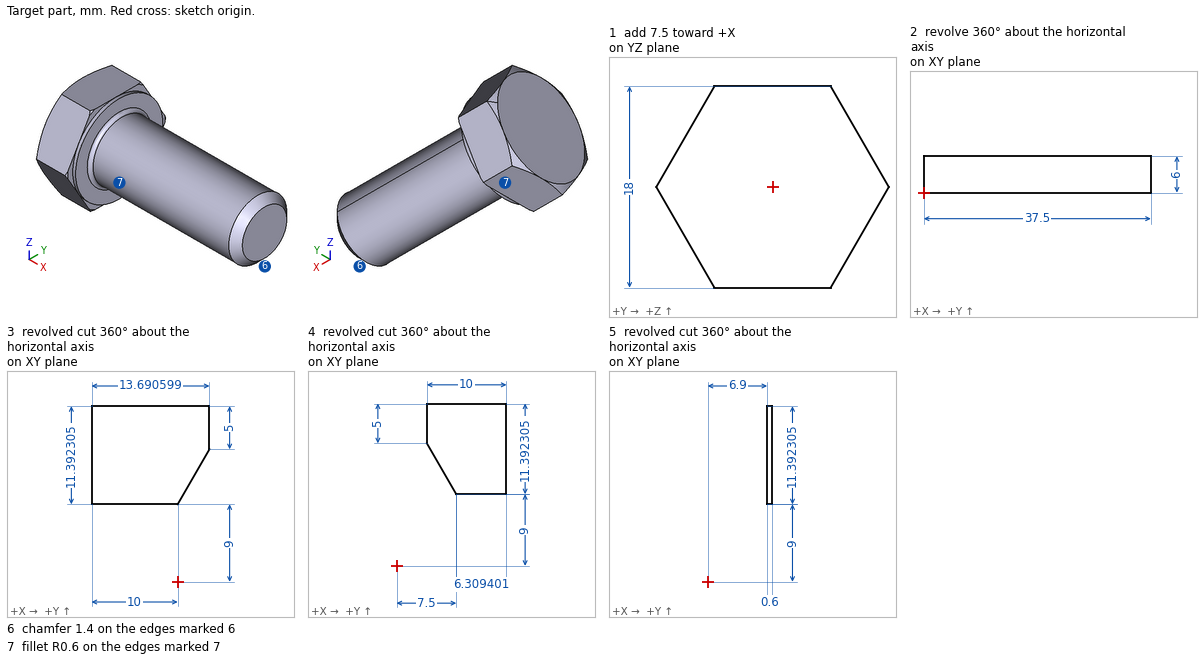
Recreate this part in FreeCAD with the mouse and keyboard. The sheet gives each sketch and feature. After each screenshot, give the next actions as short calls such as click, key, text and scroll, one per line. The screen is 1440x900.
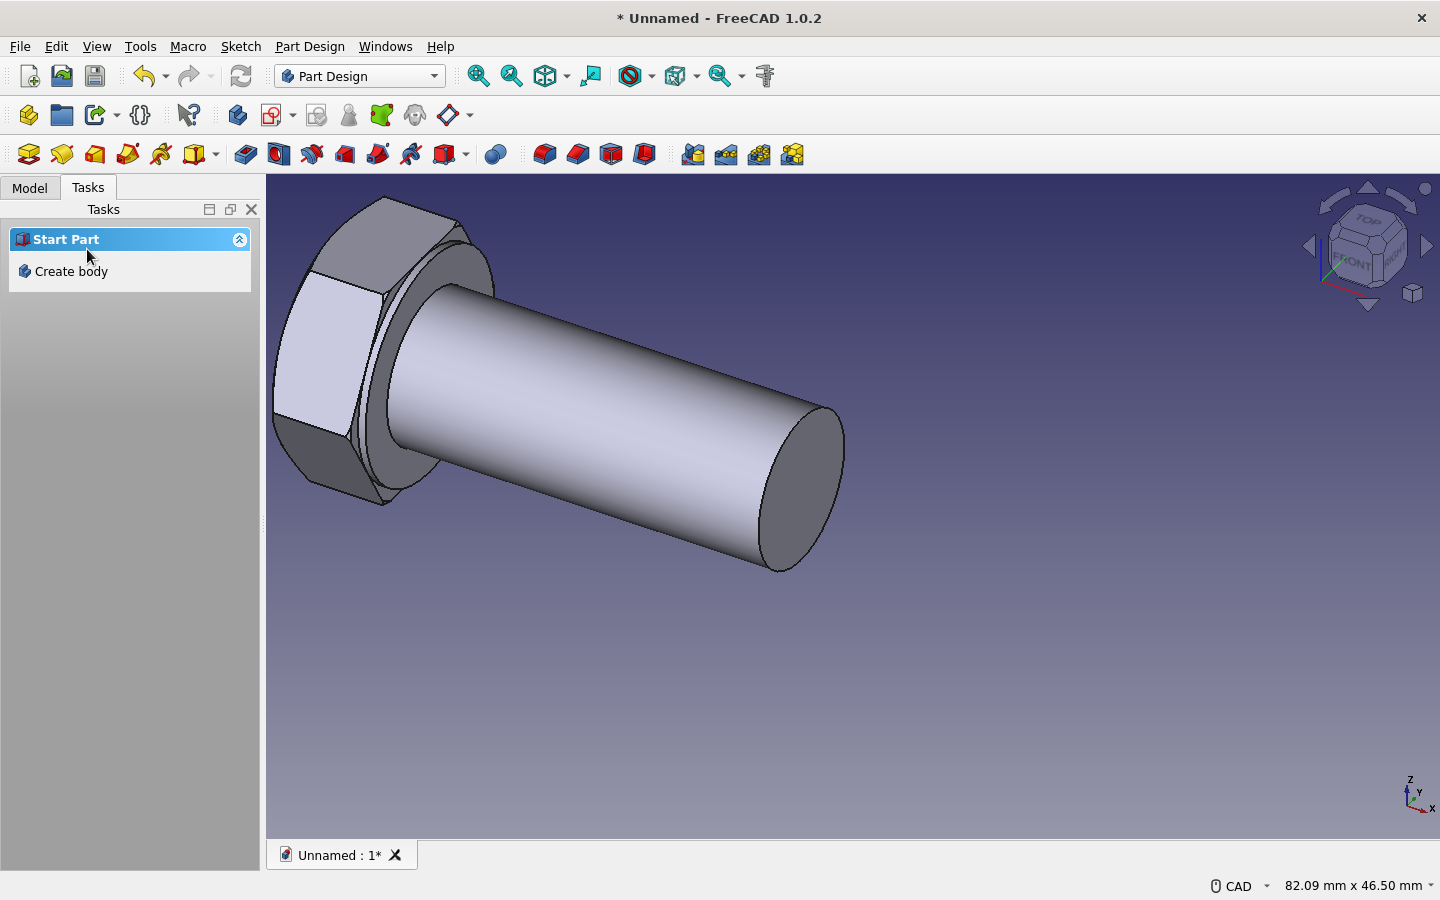
click(479, 76)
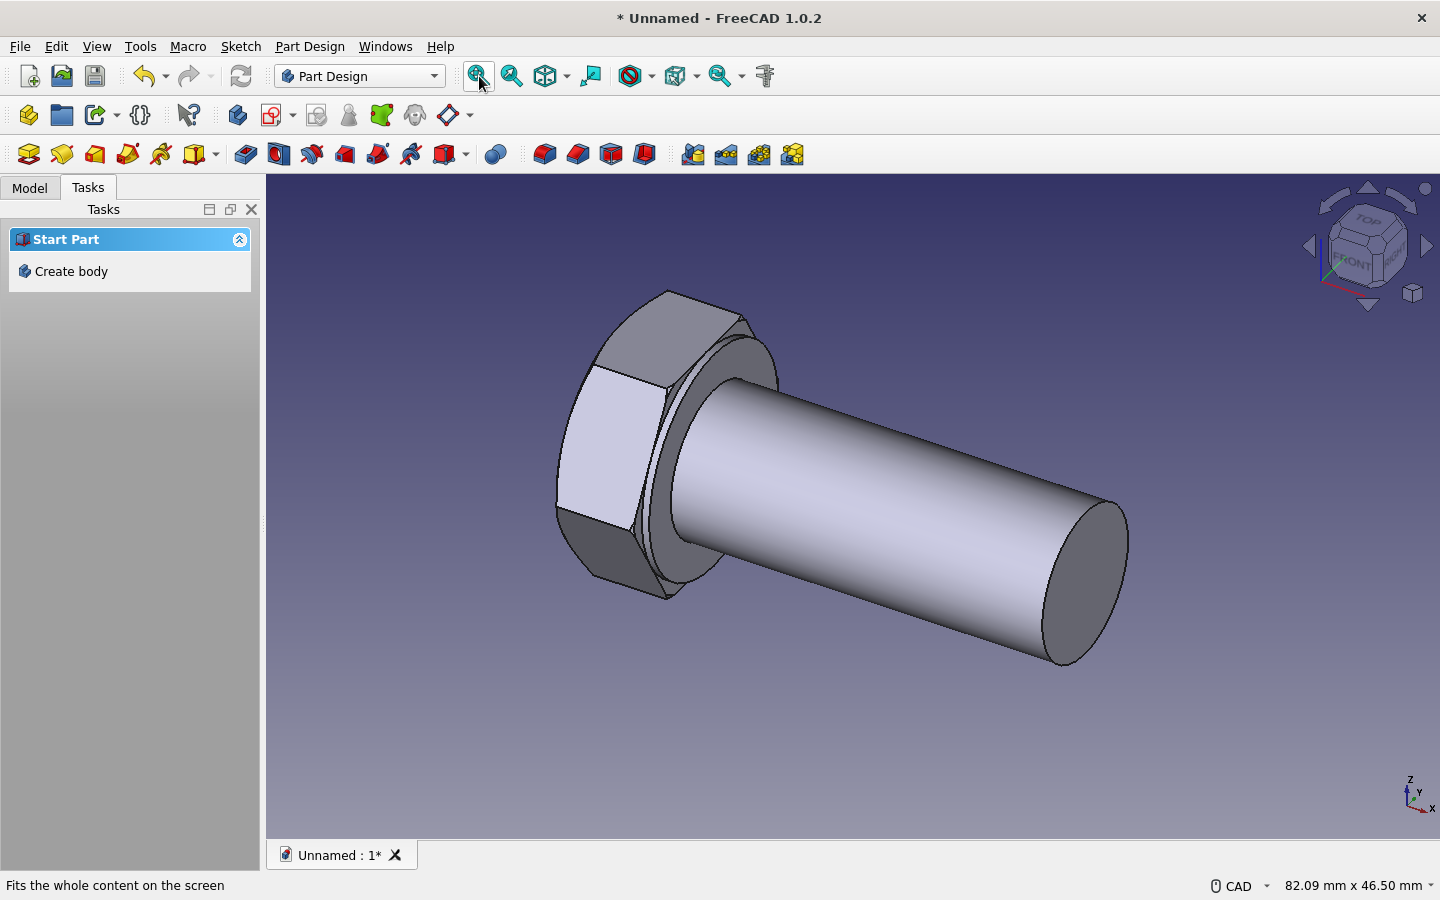
click(1042, 625)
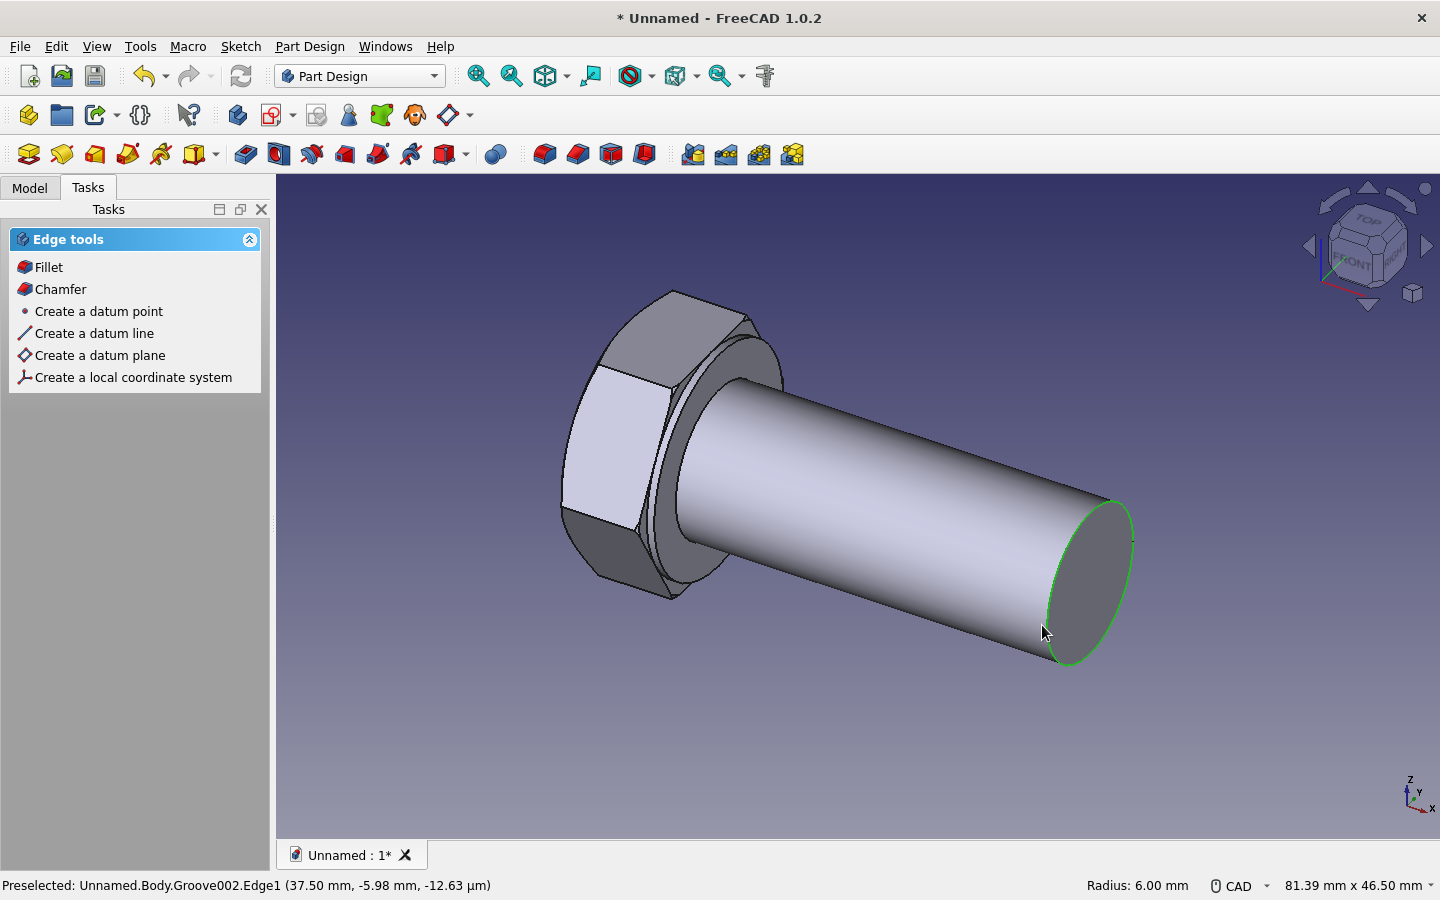
click(578, 154)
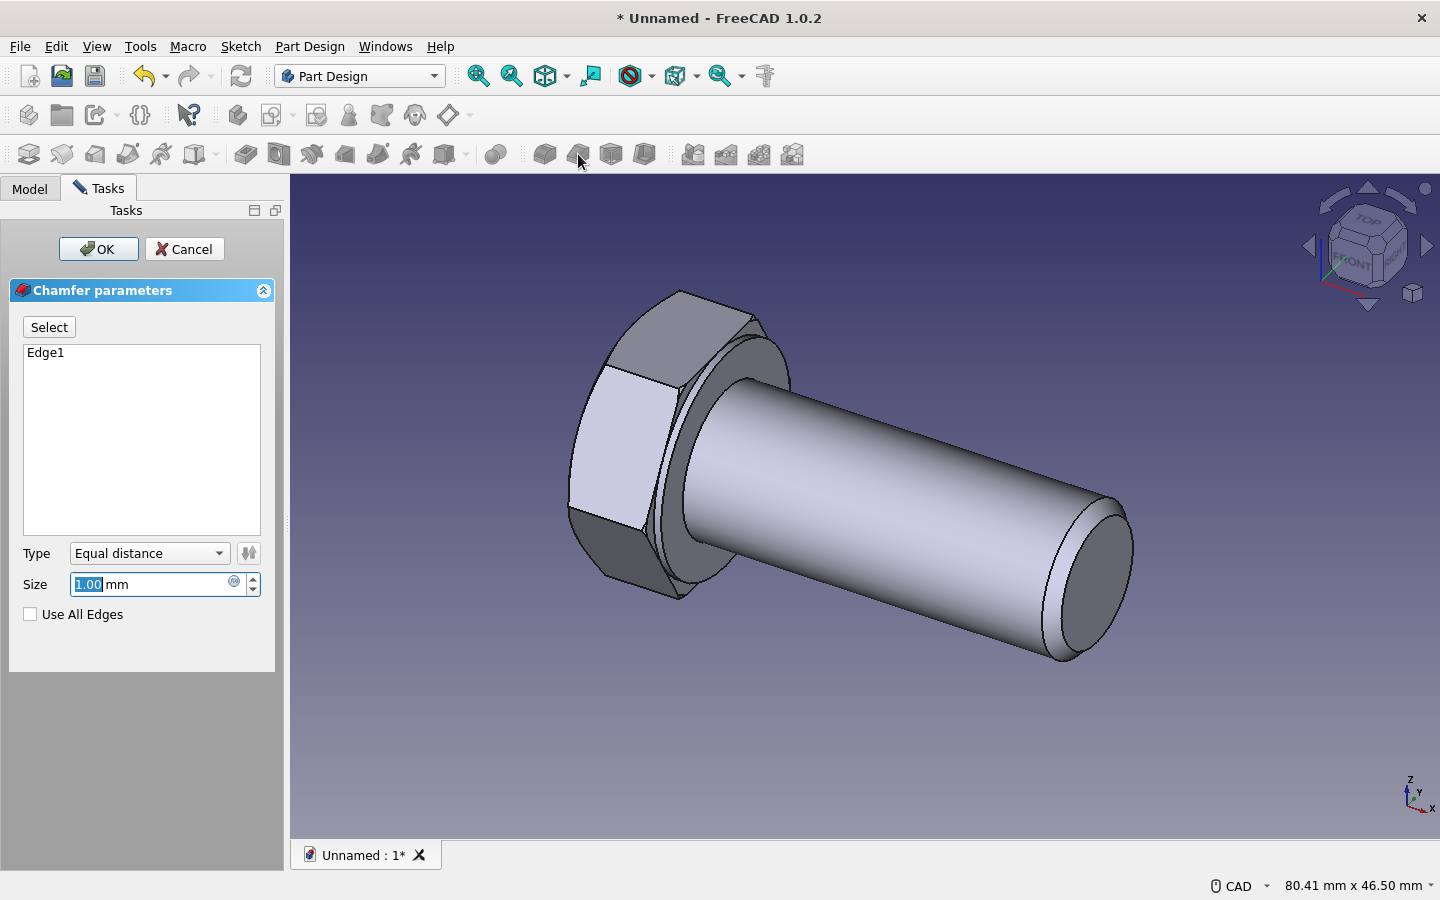
text(1.4)
key(Tab)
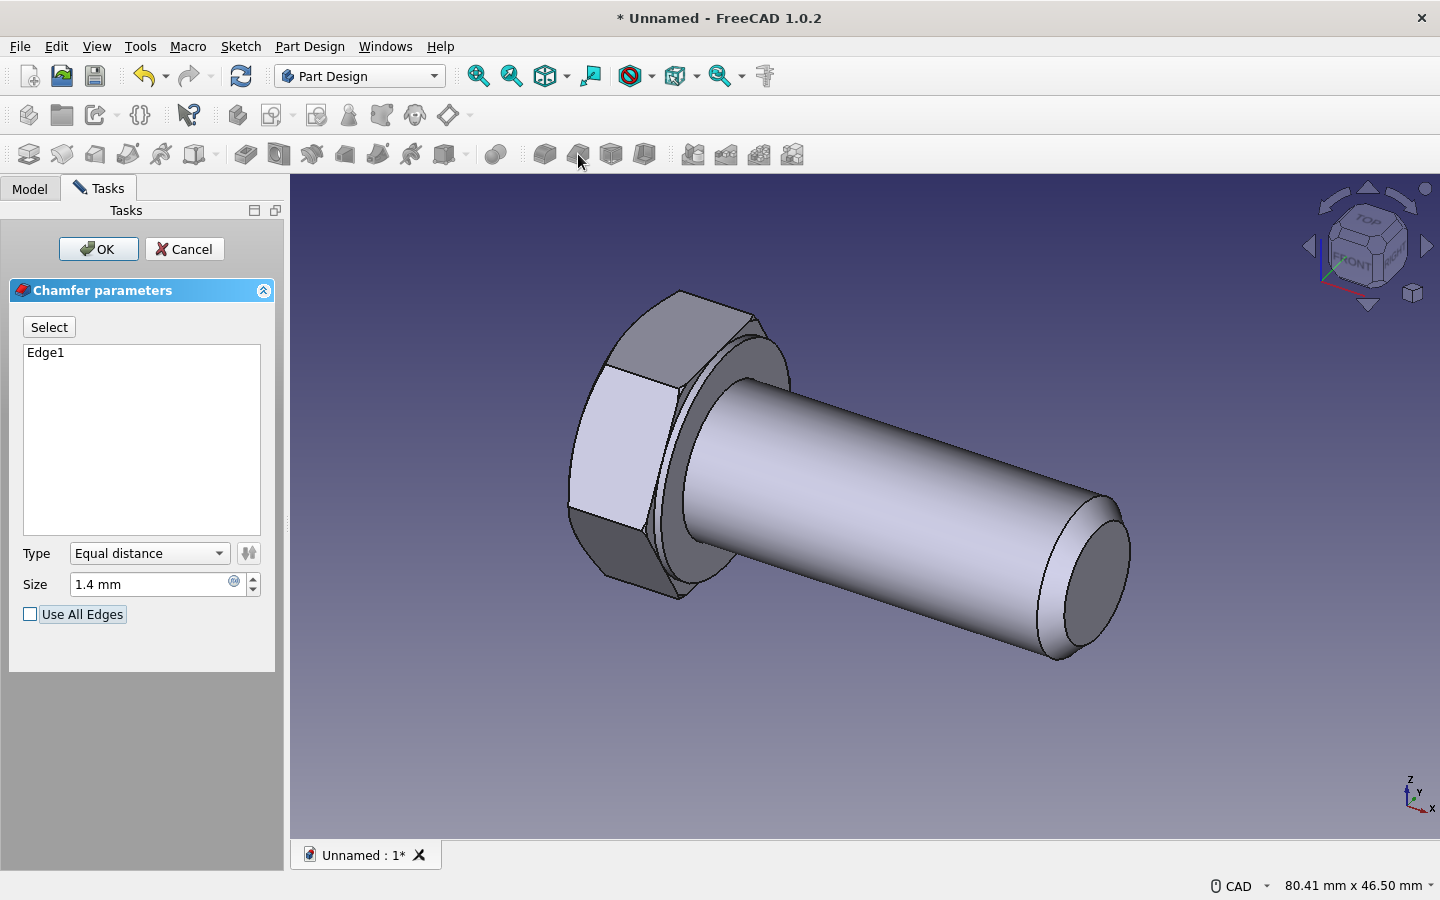
click(99, 249)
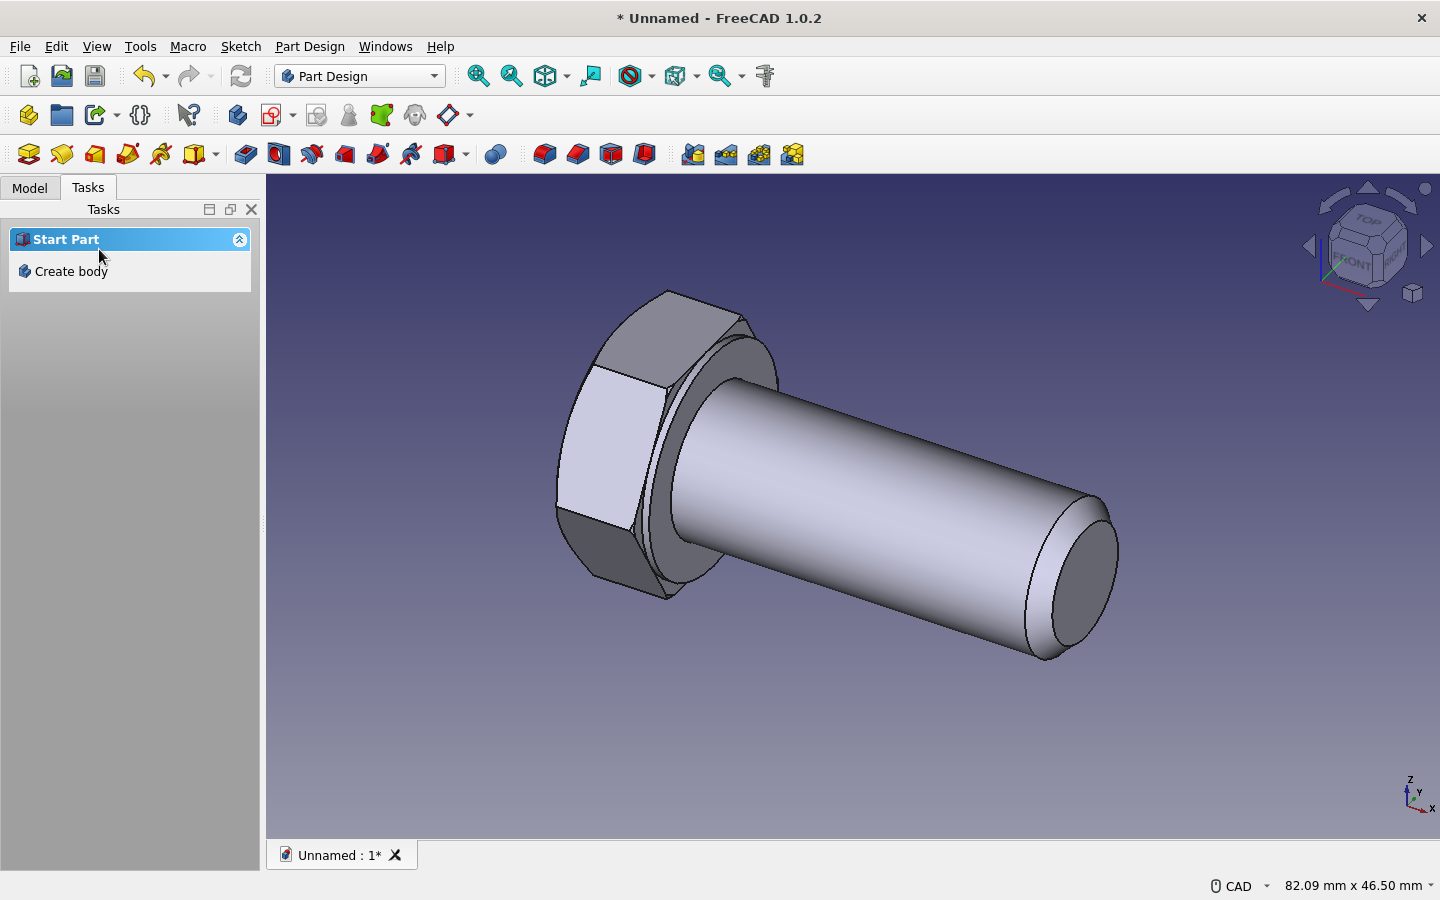
key(0)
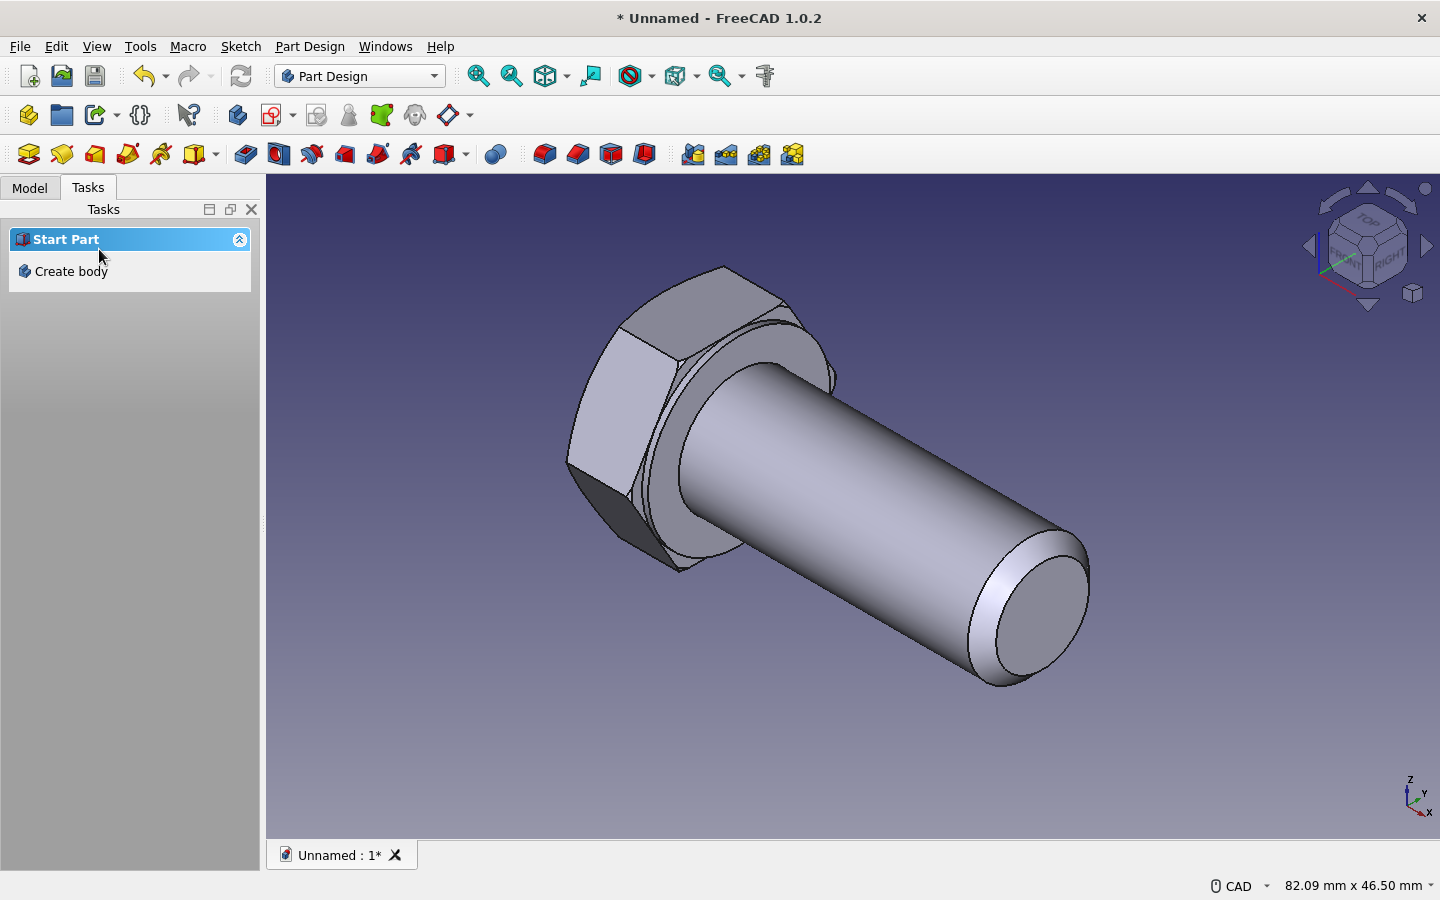
key(2)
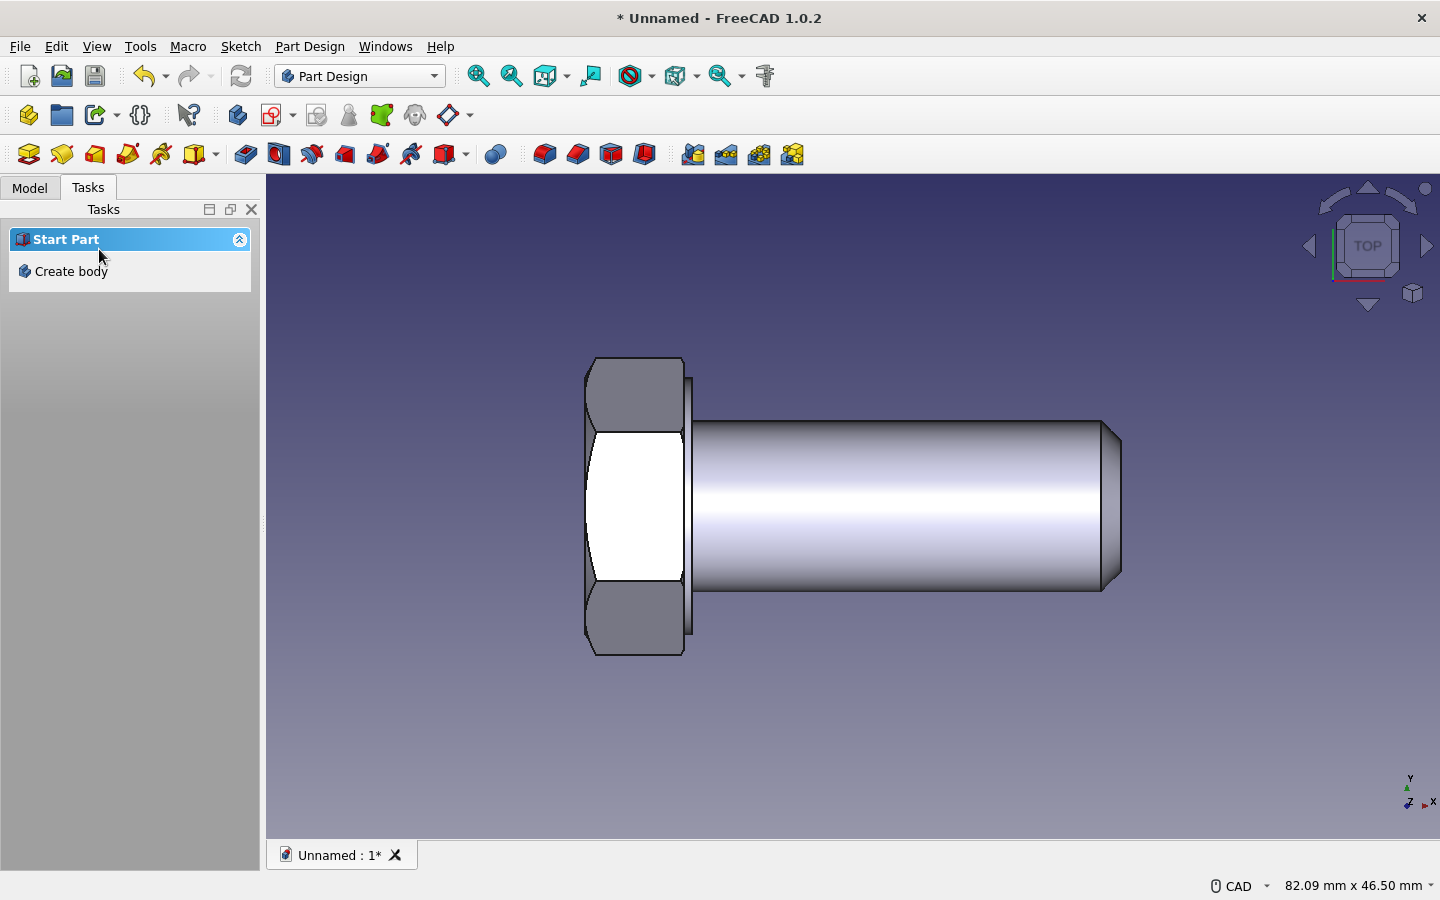
key(1)